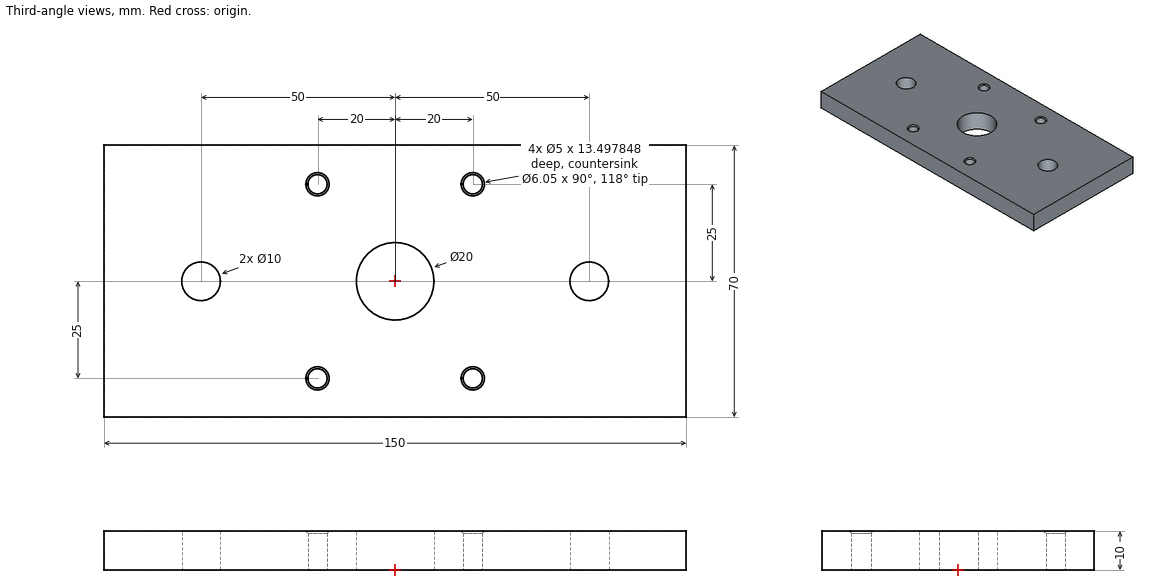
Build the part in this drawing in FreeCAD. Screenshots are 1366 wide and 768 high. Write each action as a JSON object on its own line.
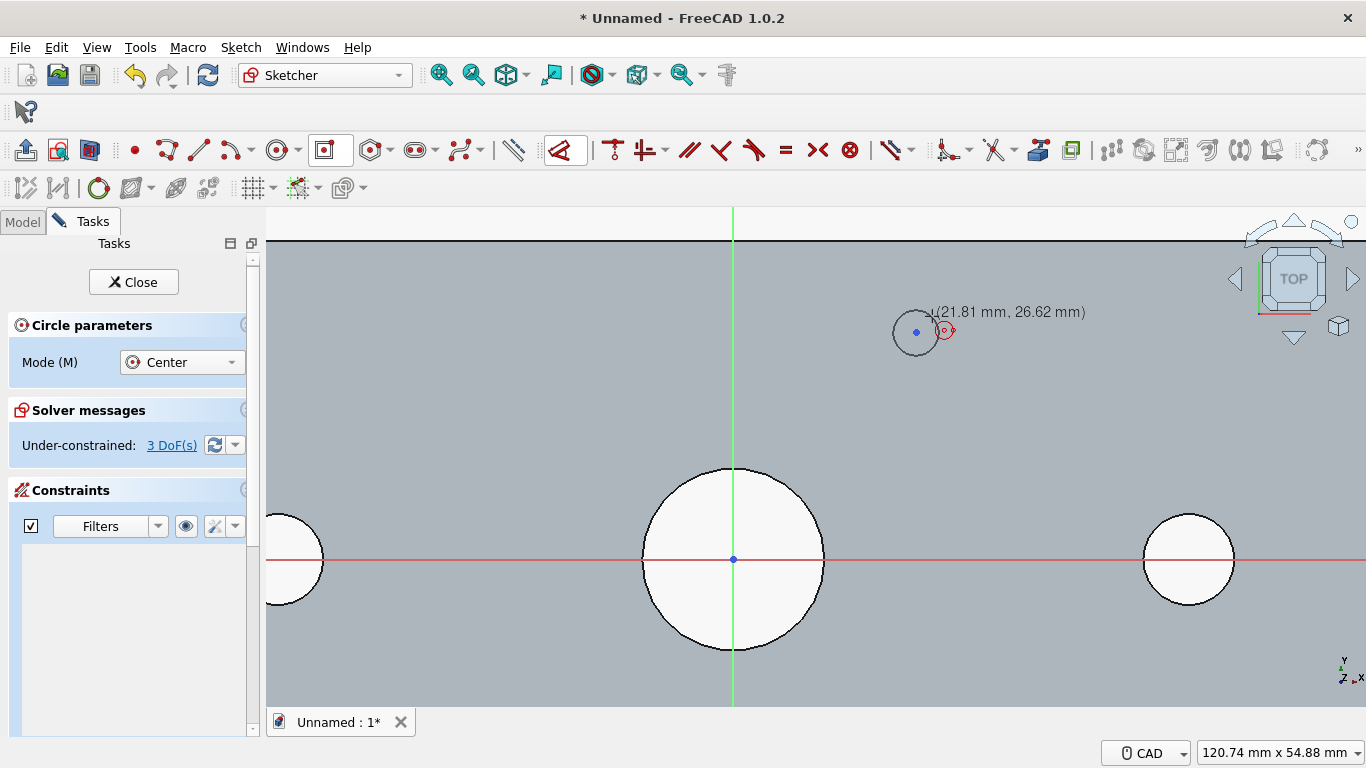
{"action": "left_click", "coordinate": [551, 332]}
{"action": "left_click", "coordinate": [567, 316]}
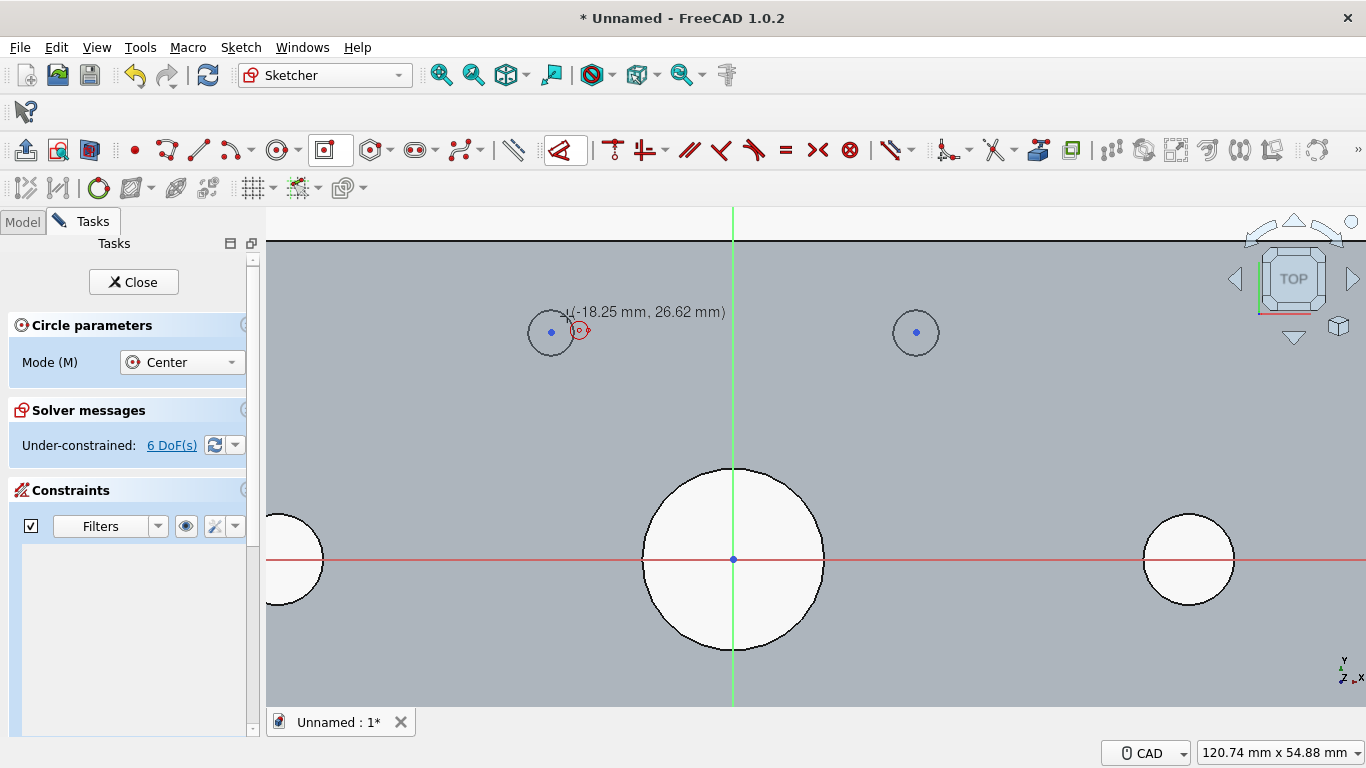
{"action": "scroll", "coordinate": [776, 248], "scroll_direction": "down", "scroll_amount": 2}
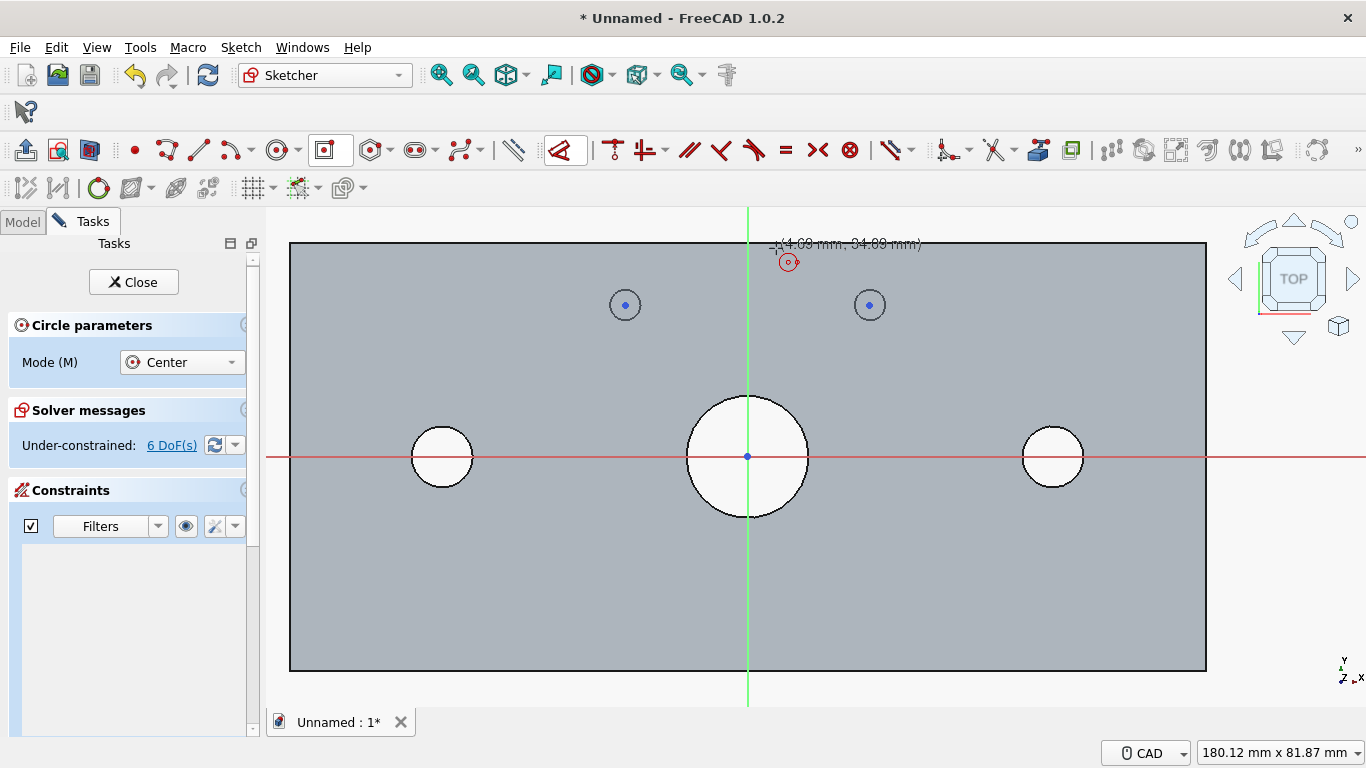
{"action": "scroll", "coordinate": [625, 610], "scroll_direction": "up", "scroll_amount": 2}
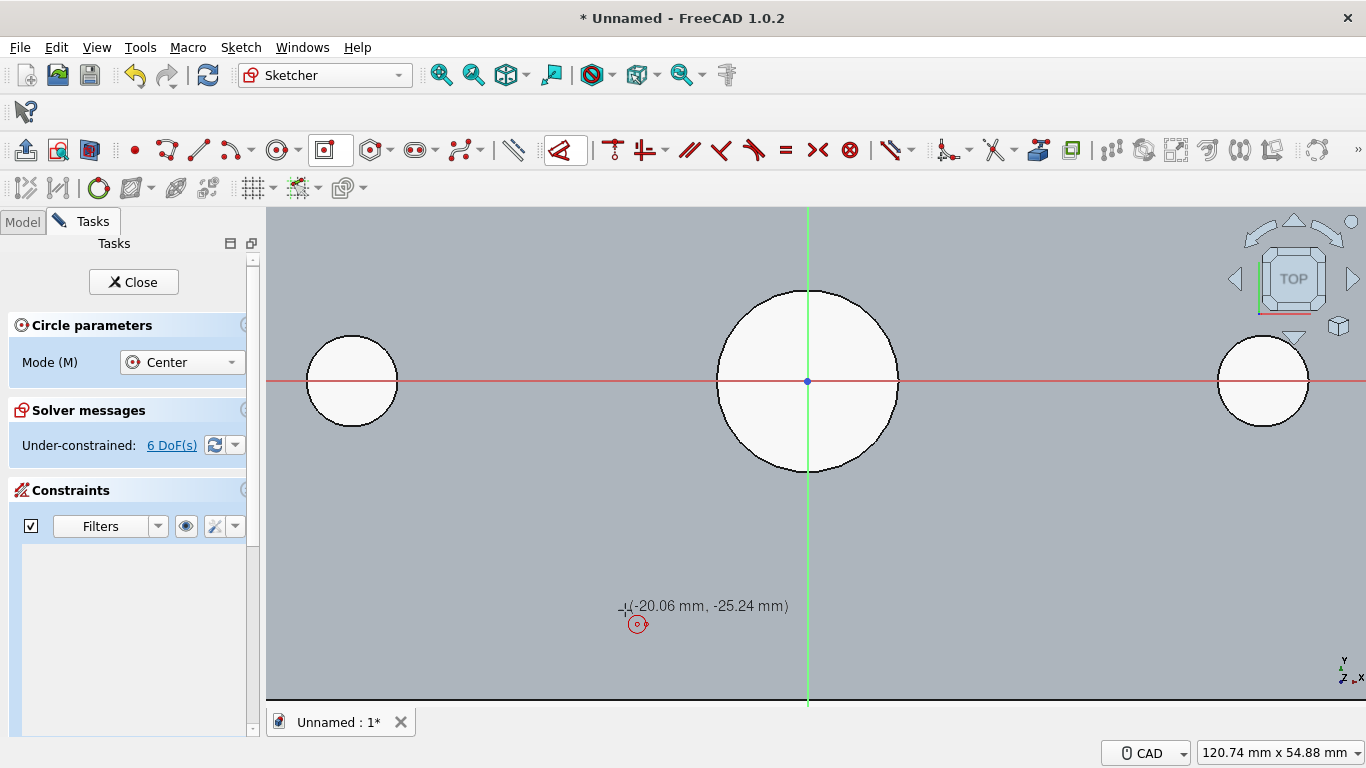
{"action": "left_click", "coordinate": [625, 609]}
{"action": "left_click", "coordinate": [642, 593]}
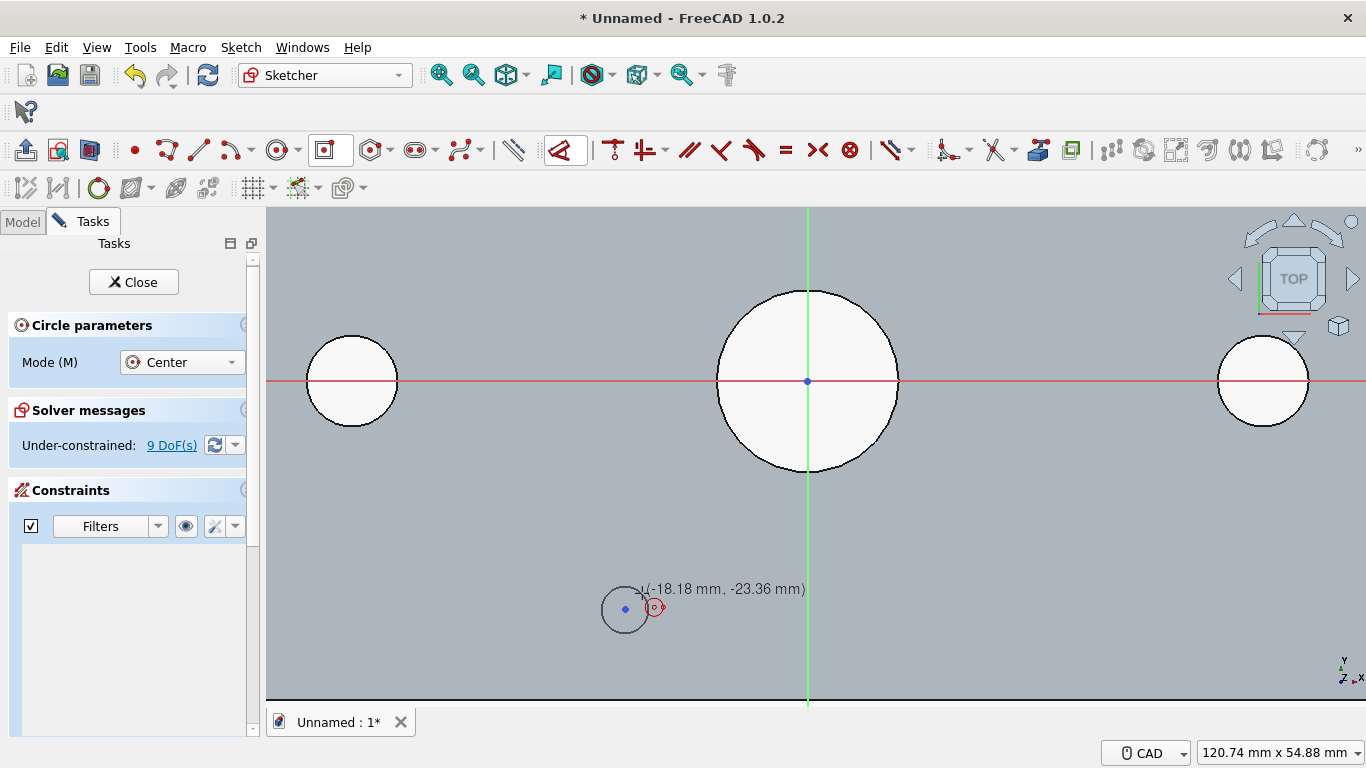
{"action": "left_click", "coordinate": [990, 609]}
{"action": "left_click", "coordinate": [1006, 593]}
{"action": "key", "text": "Escape"}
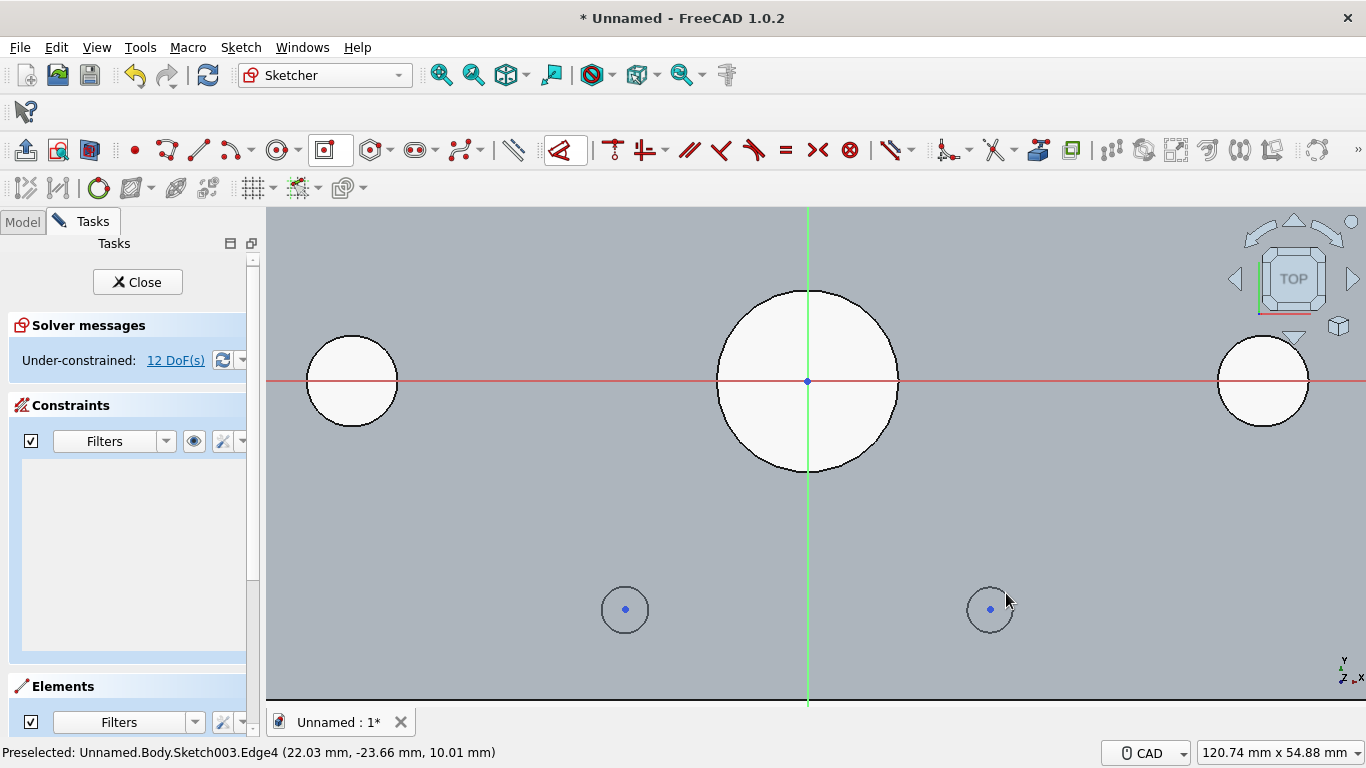
{"action": "scroll", "coordinate": [625, 611], "scroll_direction": "down", "scroll_amount": 2}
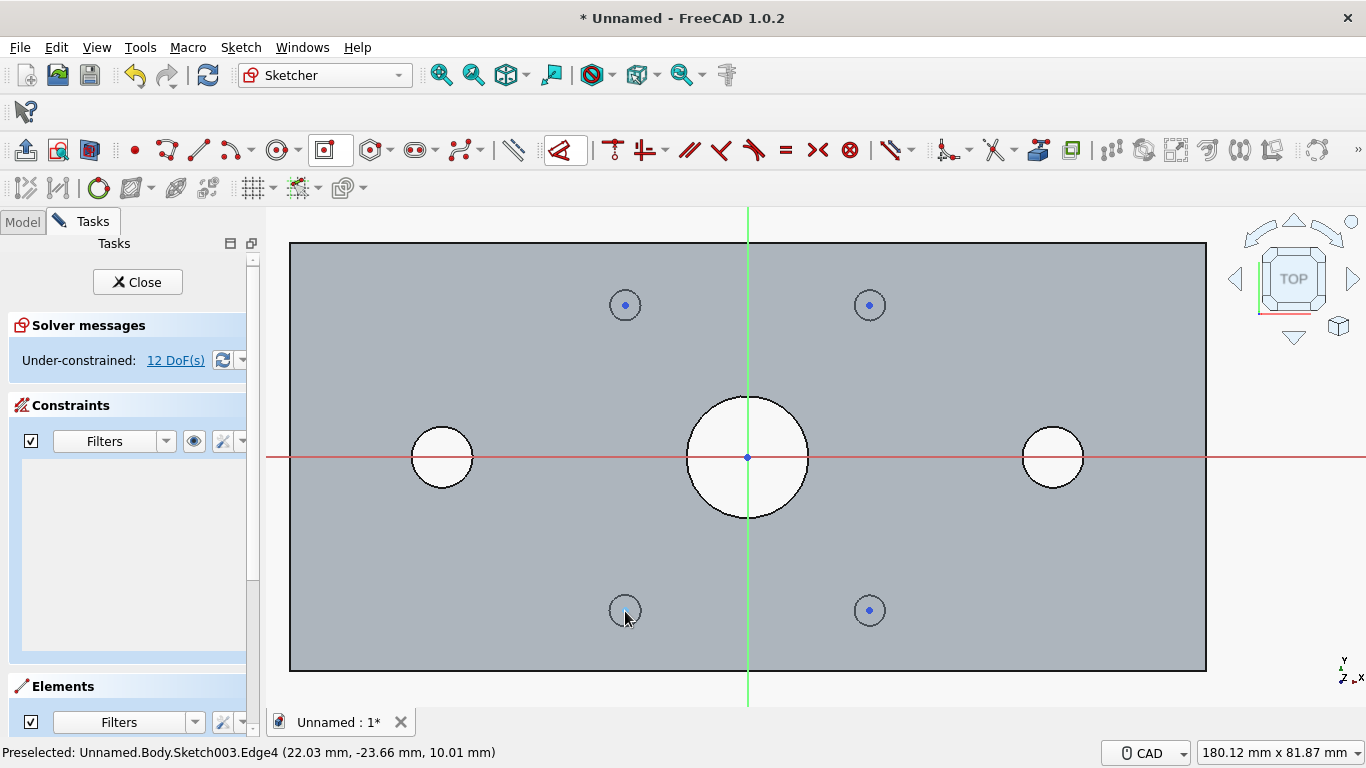
{"action": "left_click", "coordinate": [881, 295]}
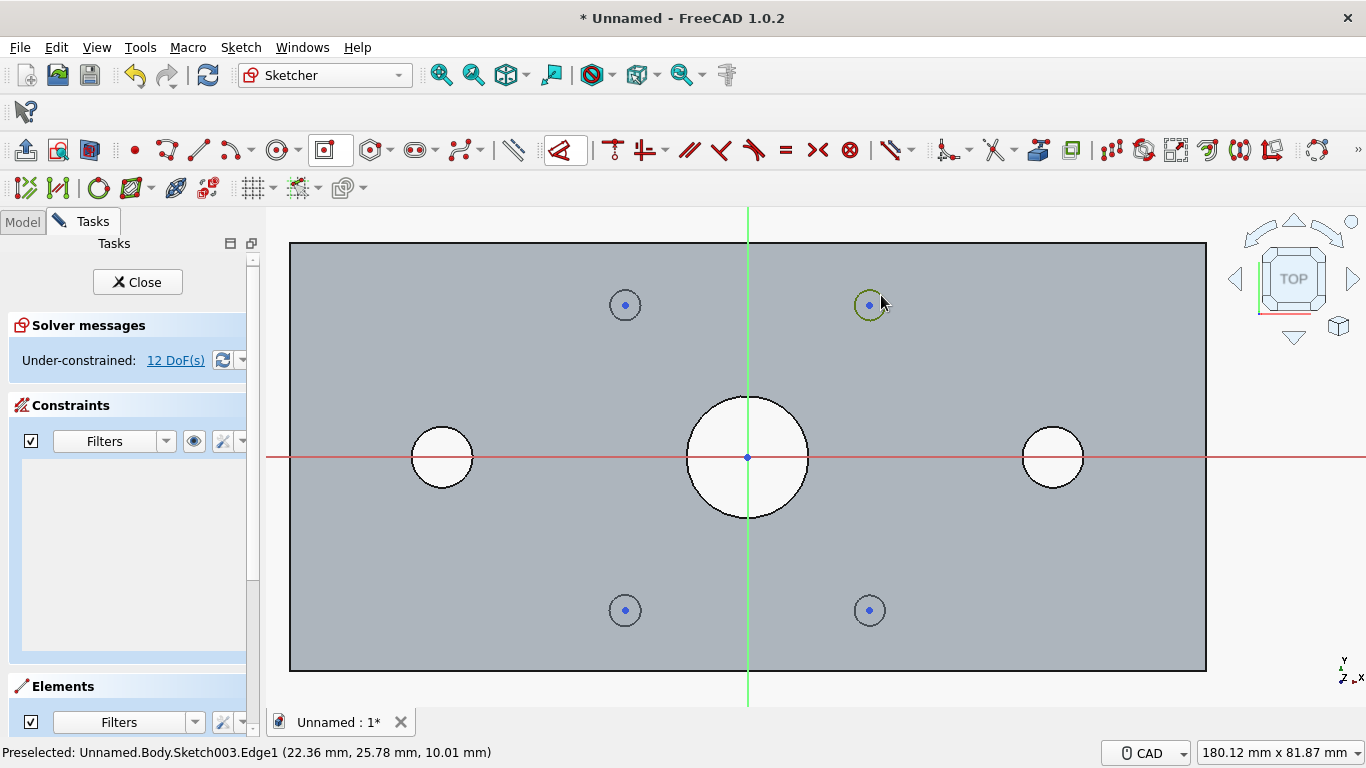
{"action": "left_click", "coordinate": [636, 295]}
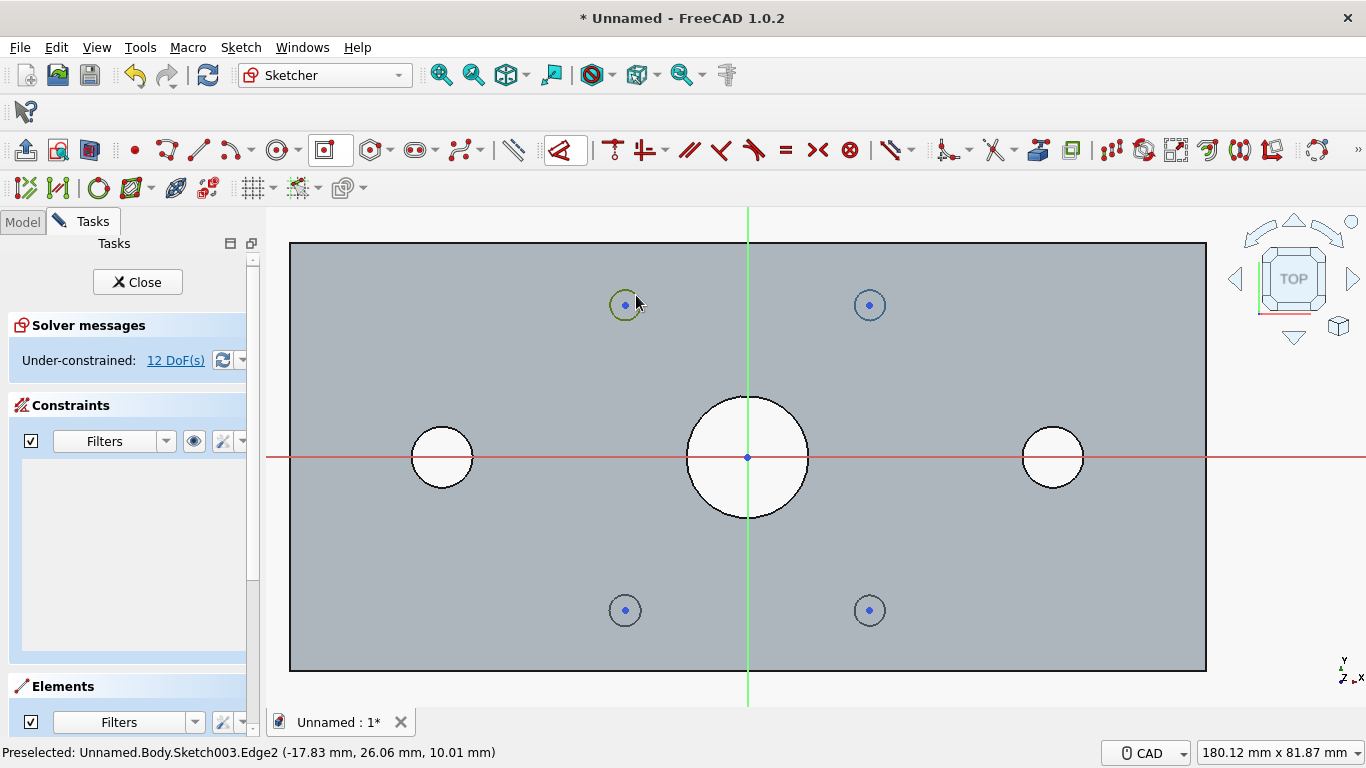
{"action": "left_click", "coordinate": [636, 599]}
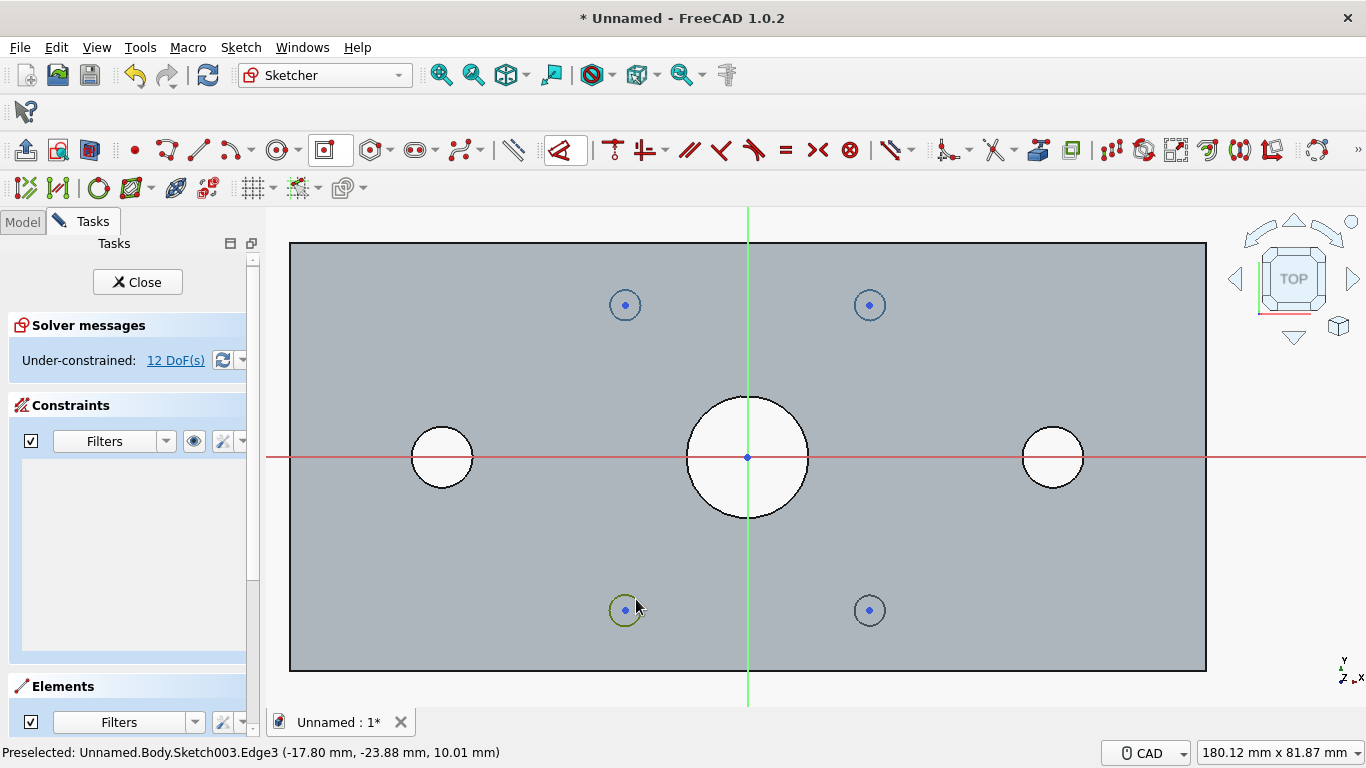
{"action": "left_click", "coordinate": [880, 600]}